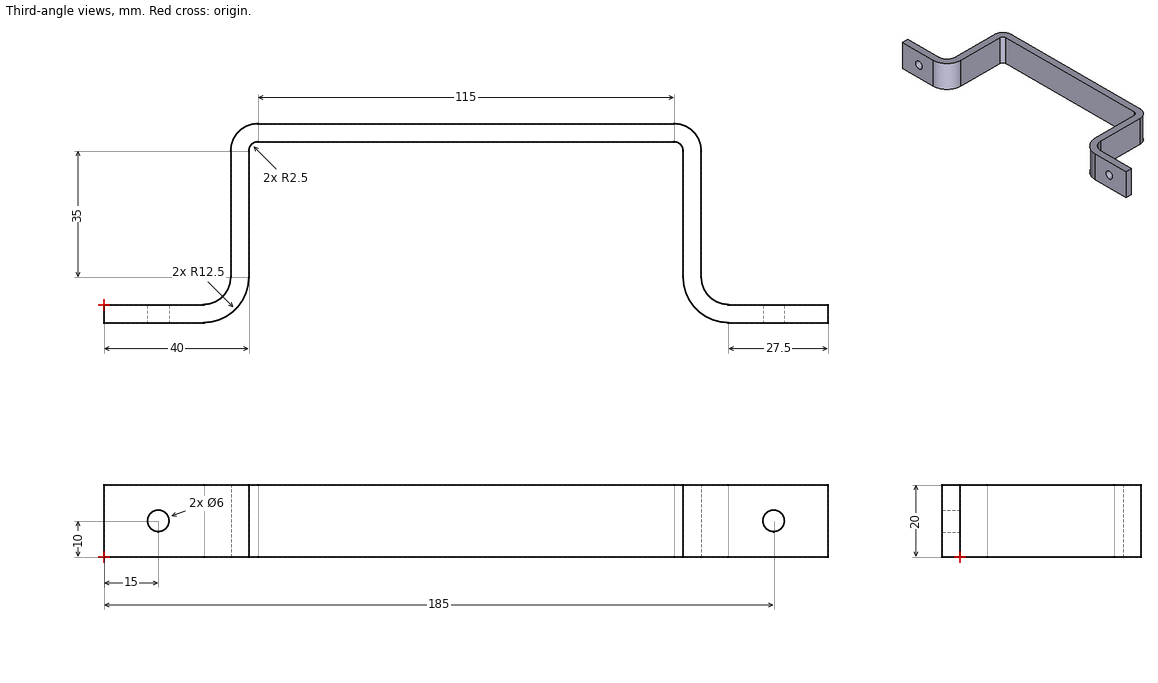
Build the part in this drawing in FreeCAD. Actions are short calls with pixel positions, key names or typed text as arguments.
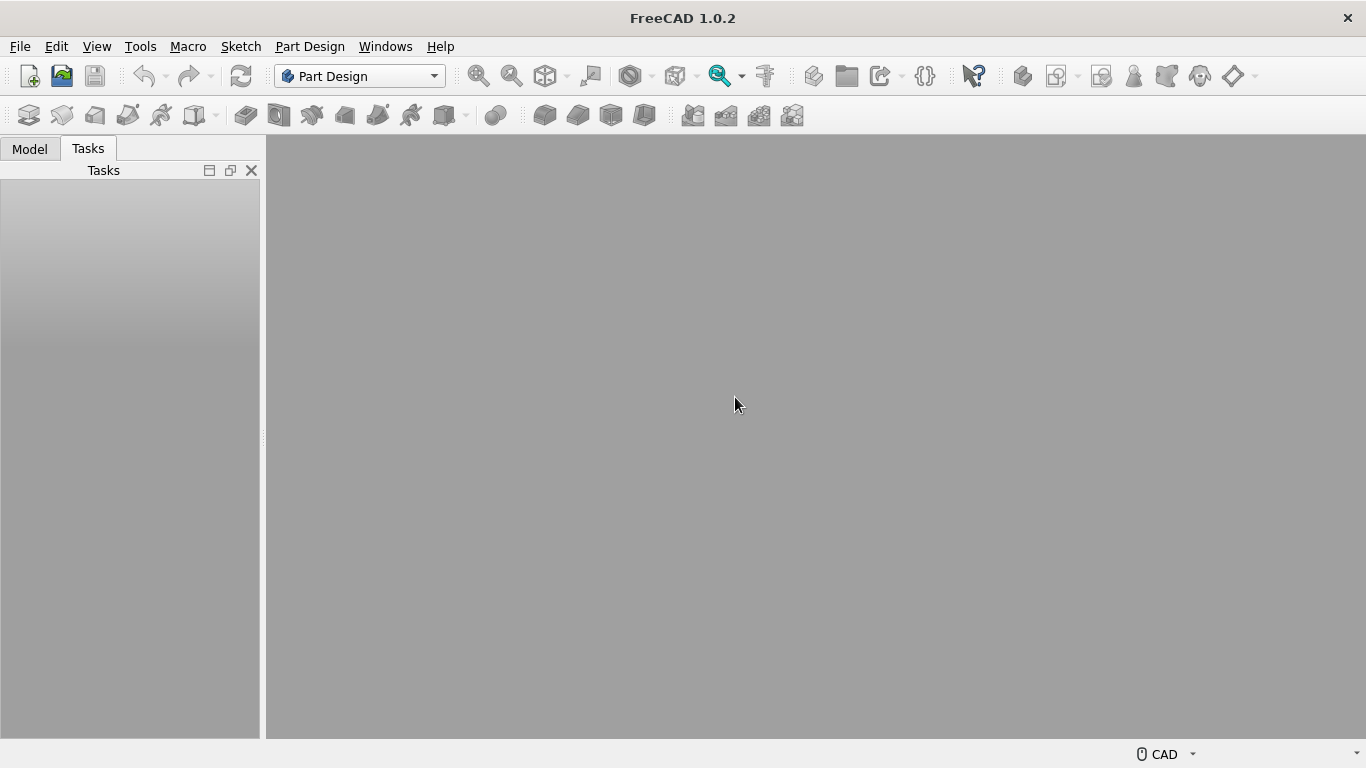
click(29, 76)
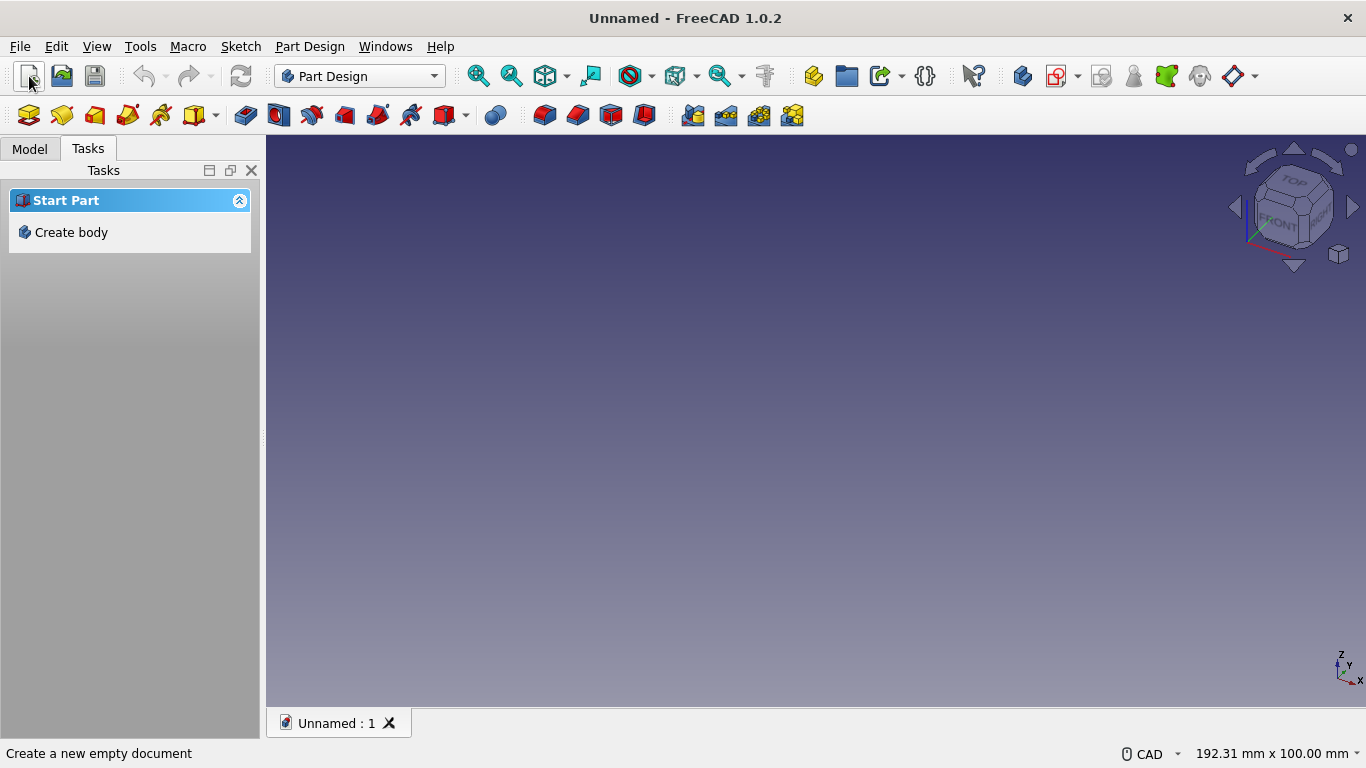
click(1056, 76)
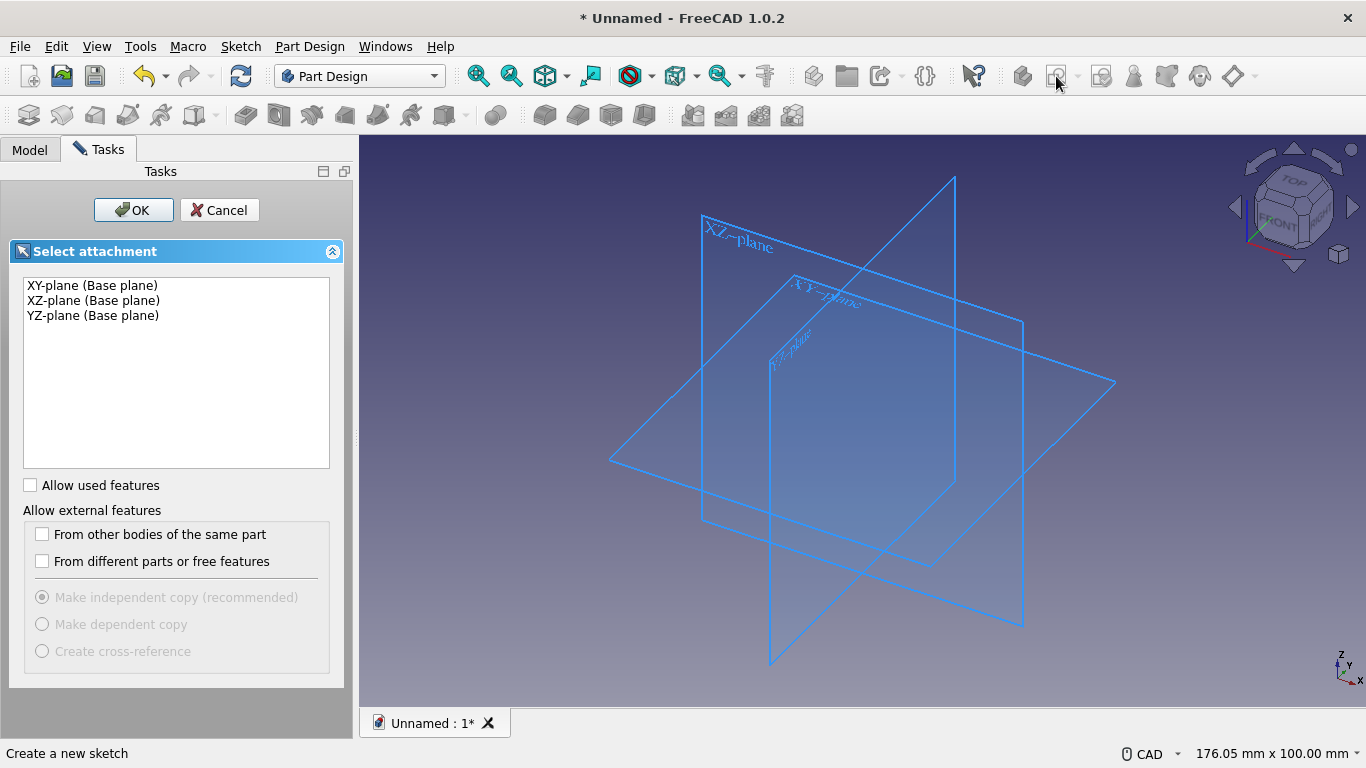
click(84, 286)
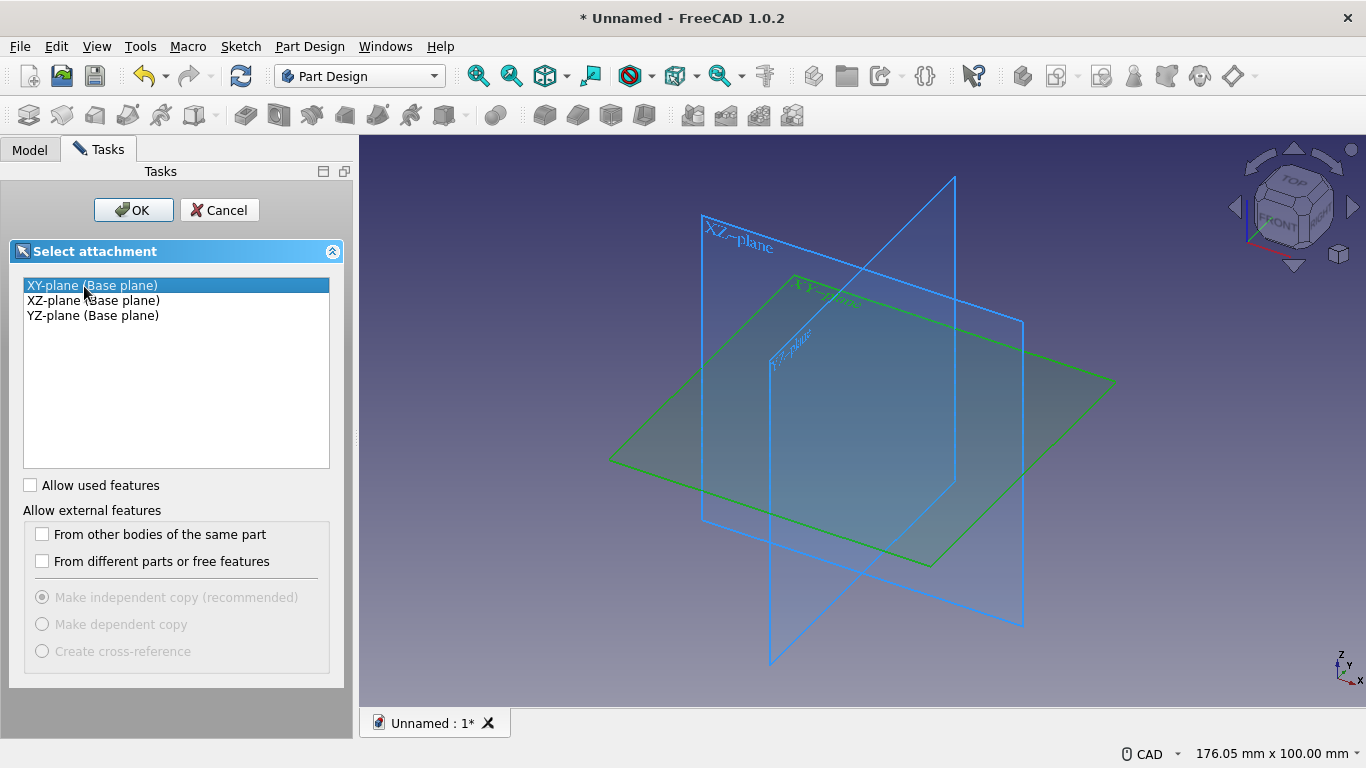
click(134, 210)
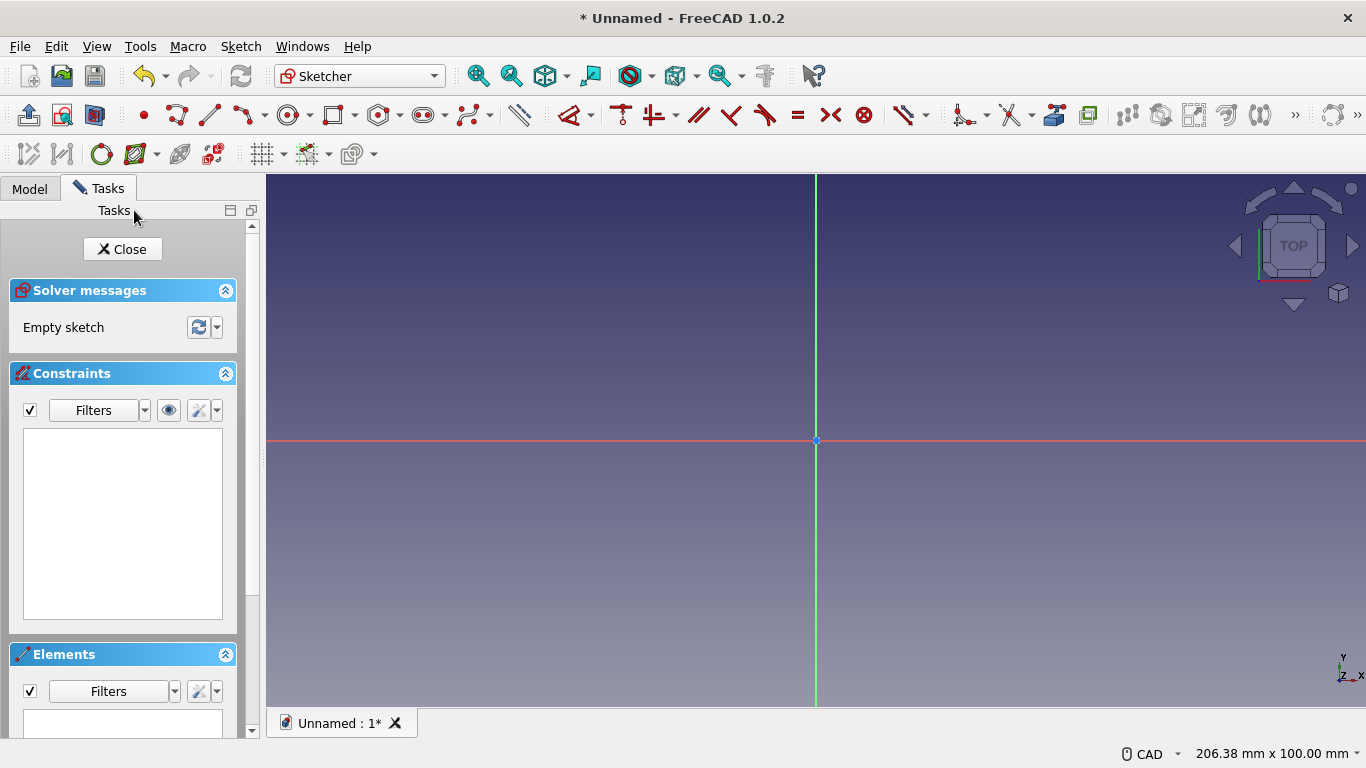
scroll(294, 586, down, 3)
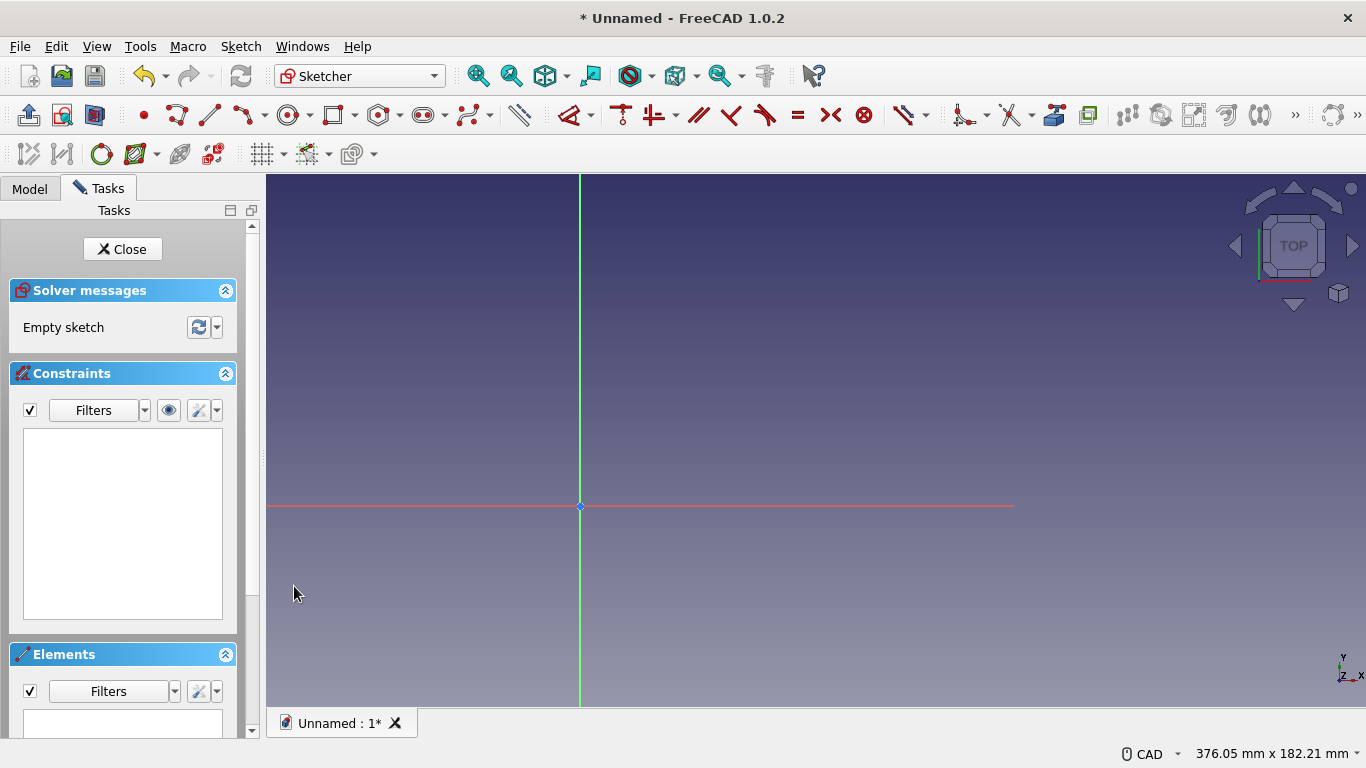
click(177, 116)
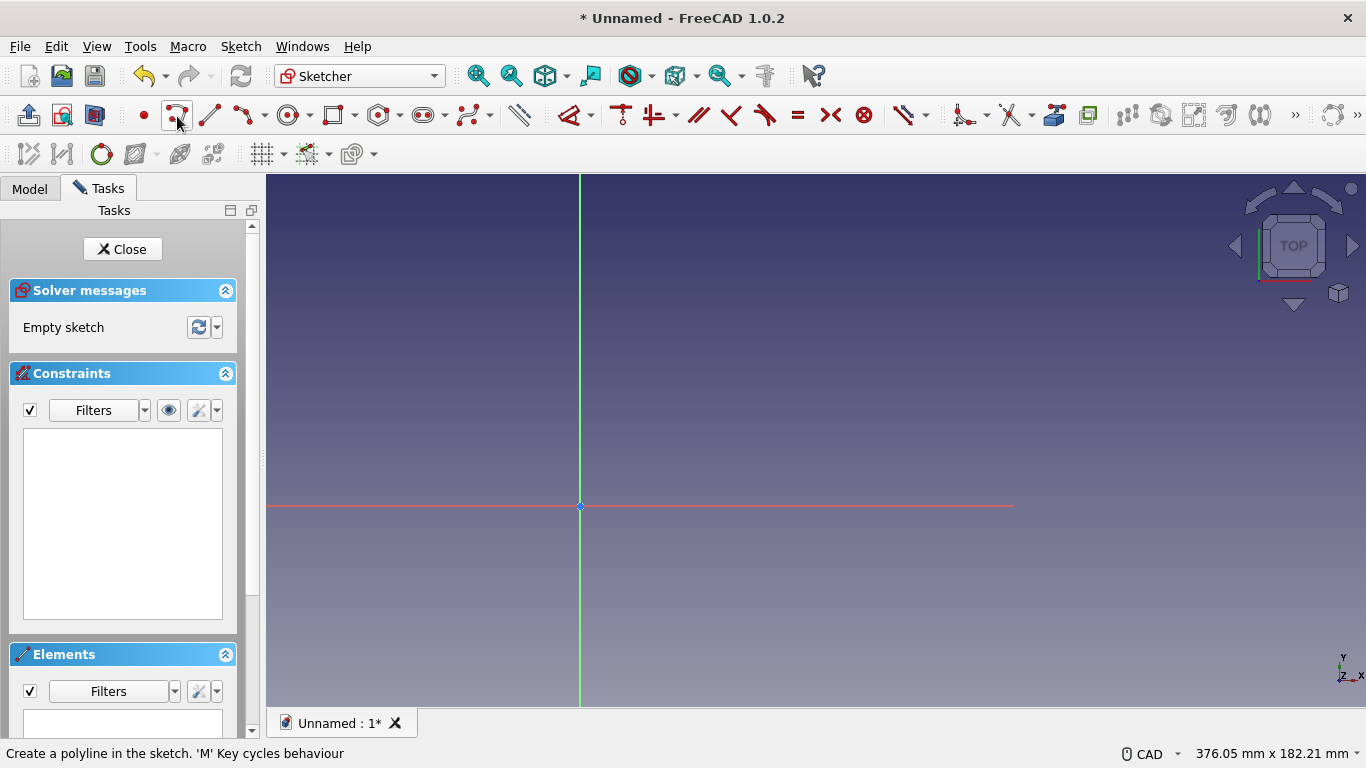
click(661, 506)
click(580, 506)
click(589, 521)
click(661, 521)
right_click(661, 521)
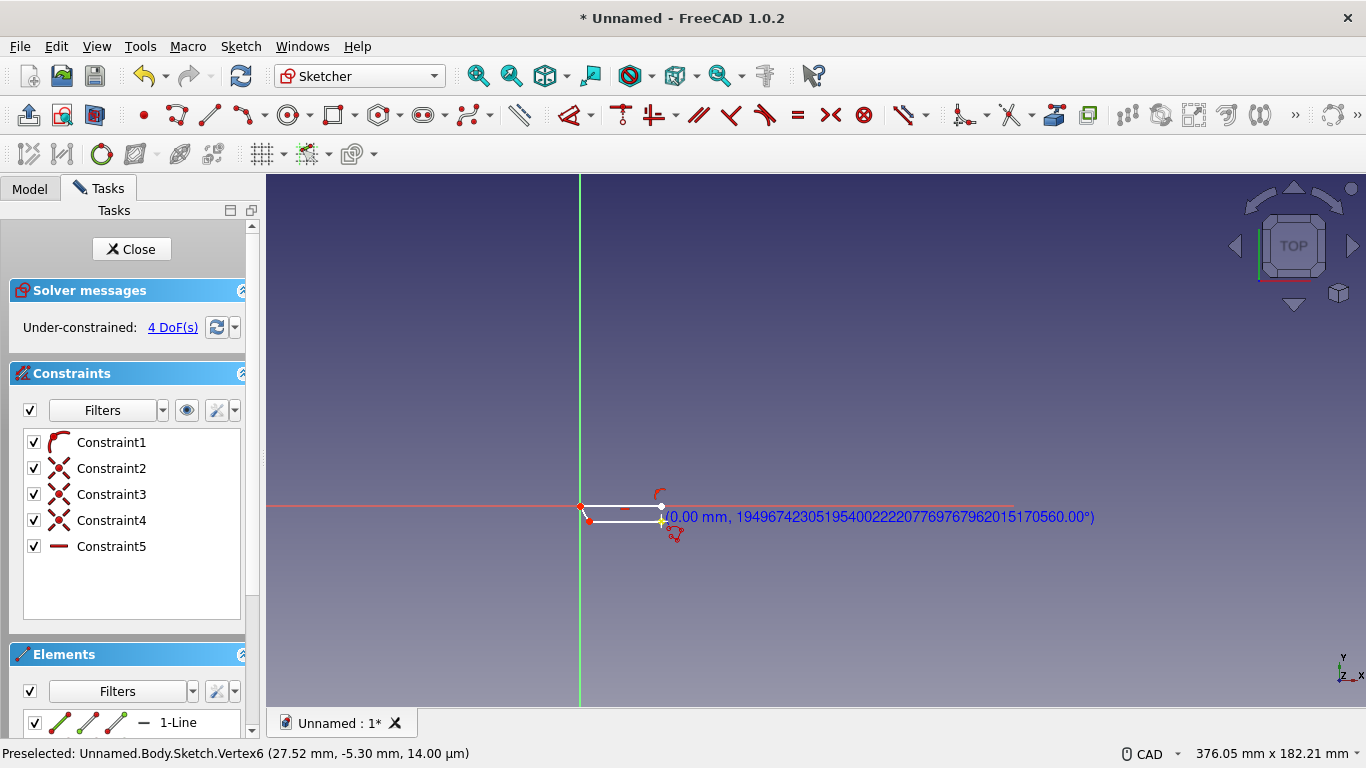
click(210, 116)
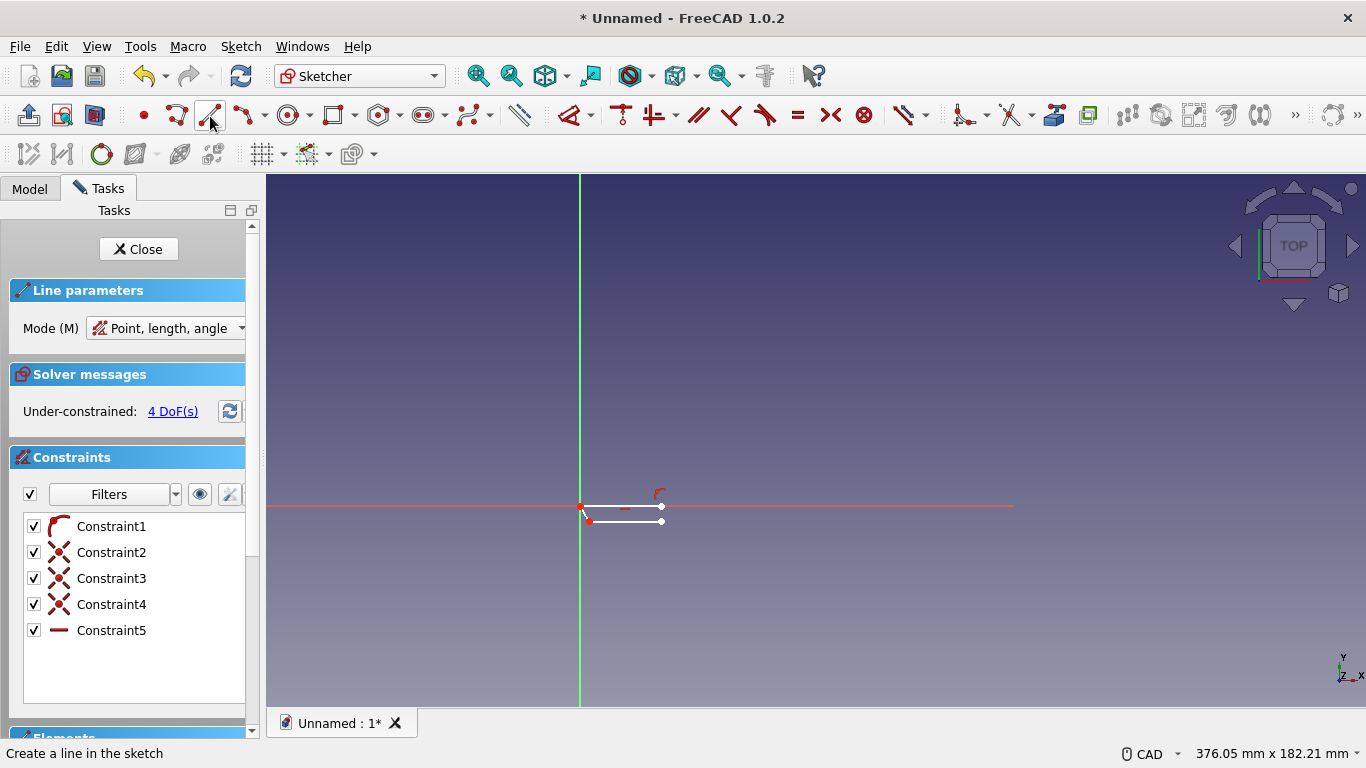
click(697, 485)
click(697, 382)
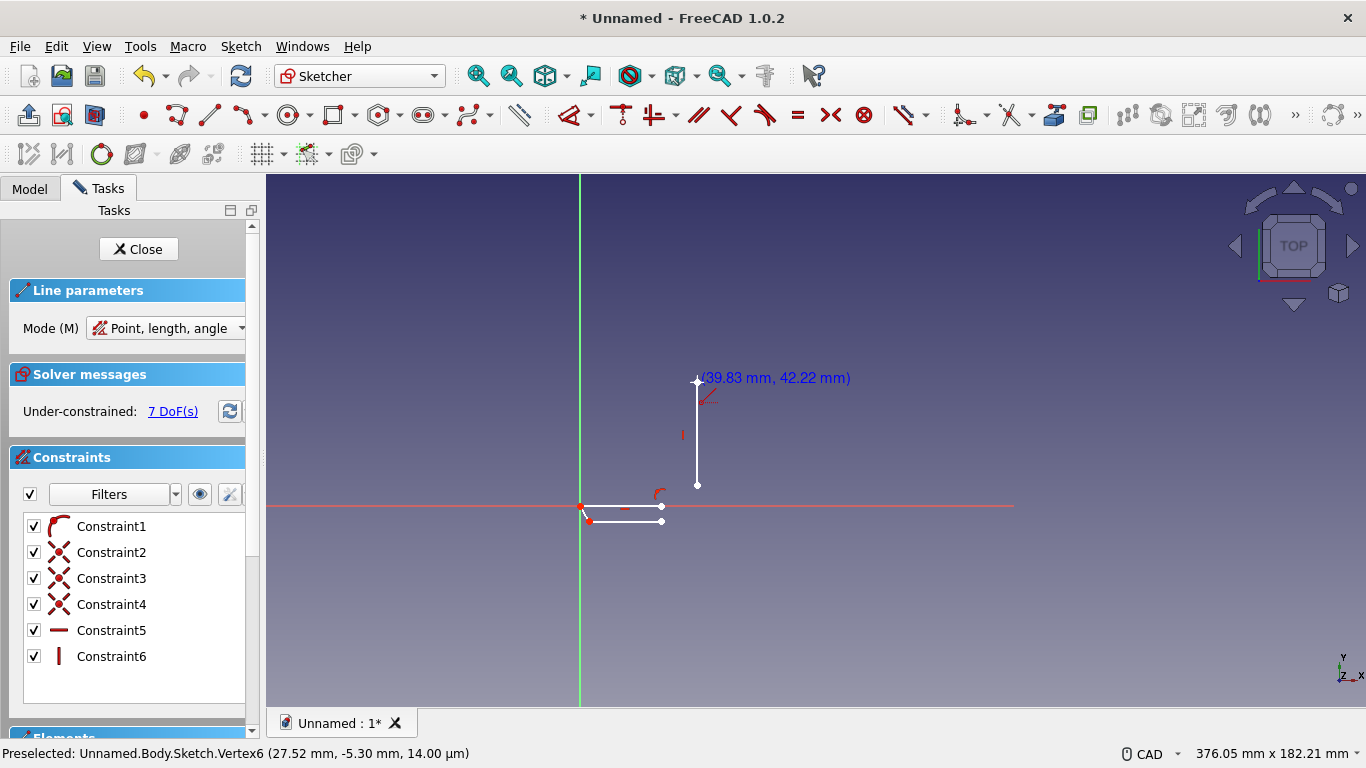
scroll(705, 375, up, 3)